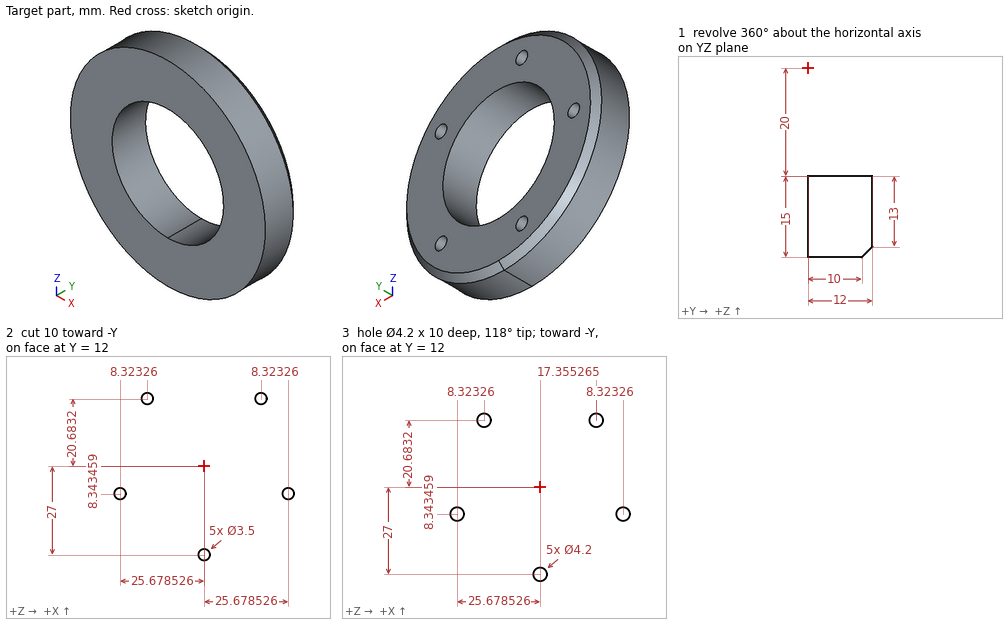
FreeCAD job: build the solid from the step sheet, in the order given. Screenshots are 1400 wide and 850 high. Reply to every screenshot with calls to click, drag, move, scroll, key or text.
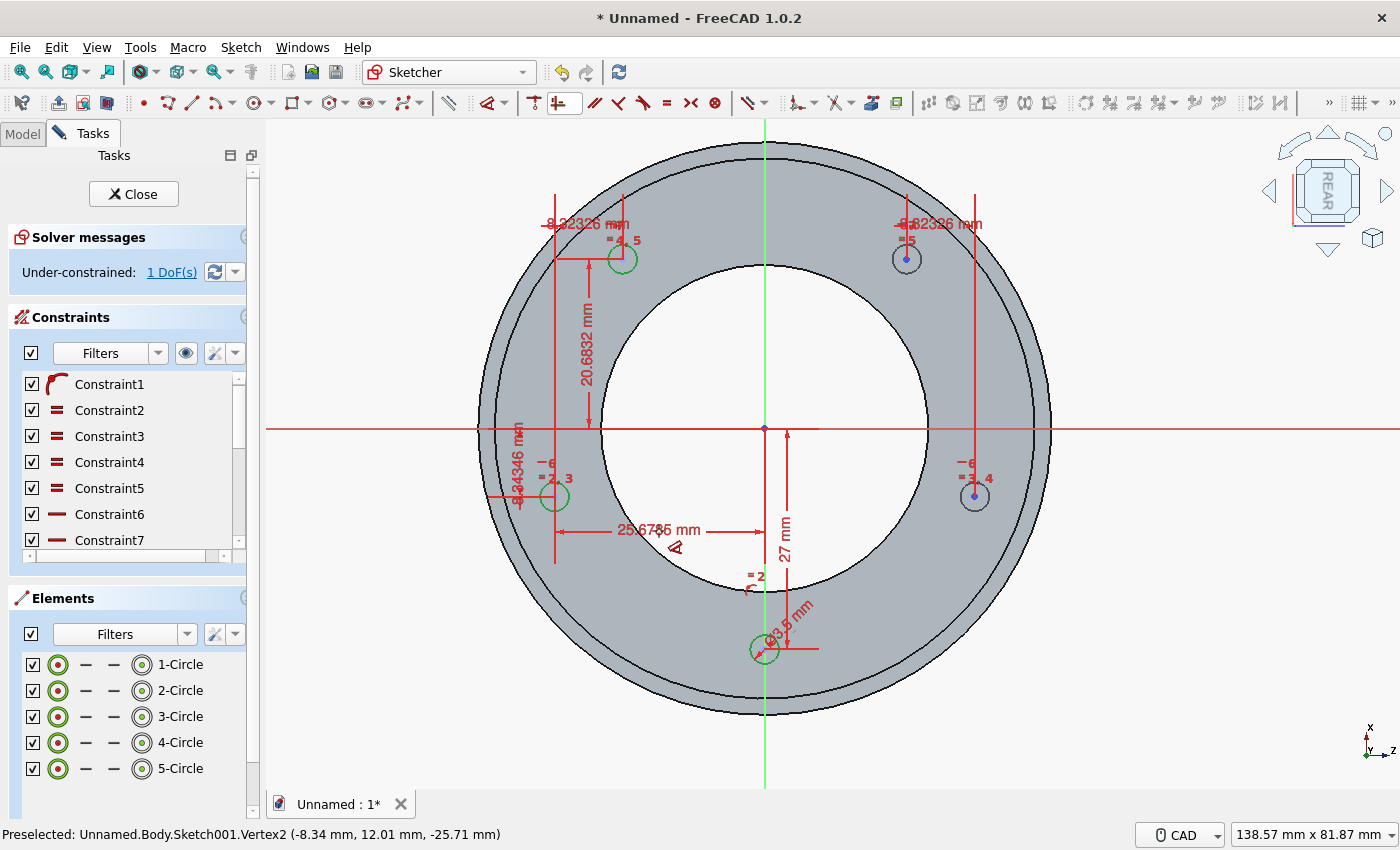
click(975, 497)
click(870, 531)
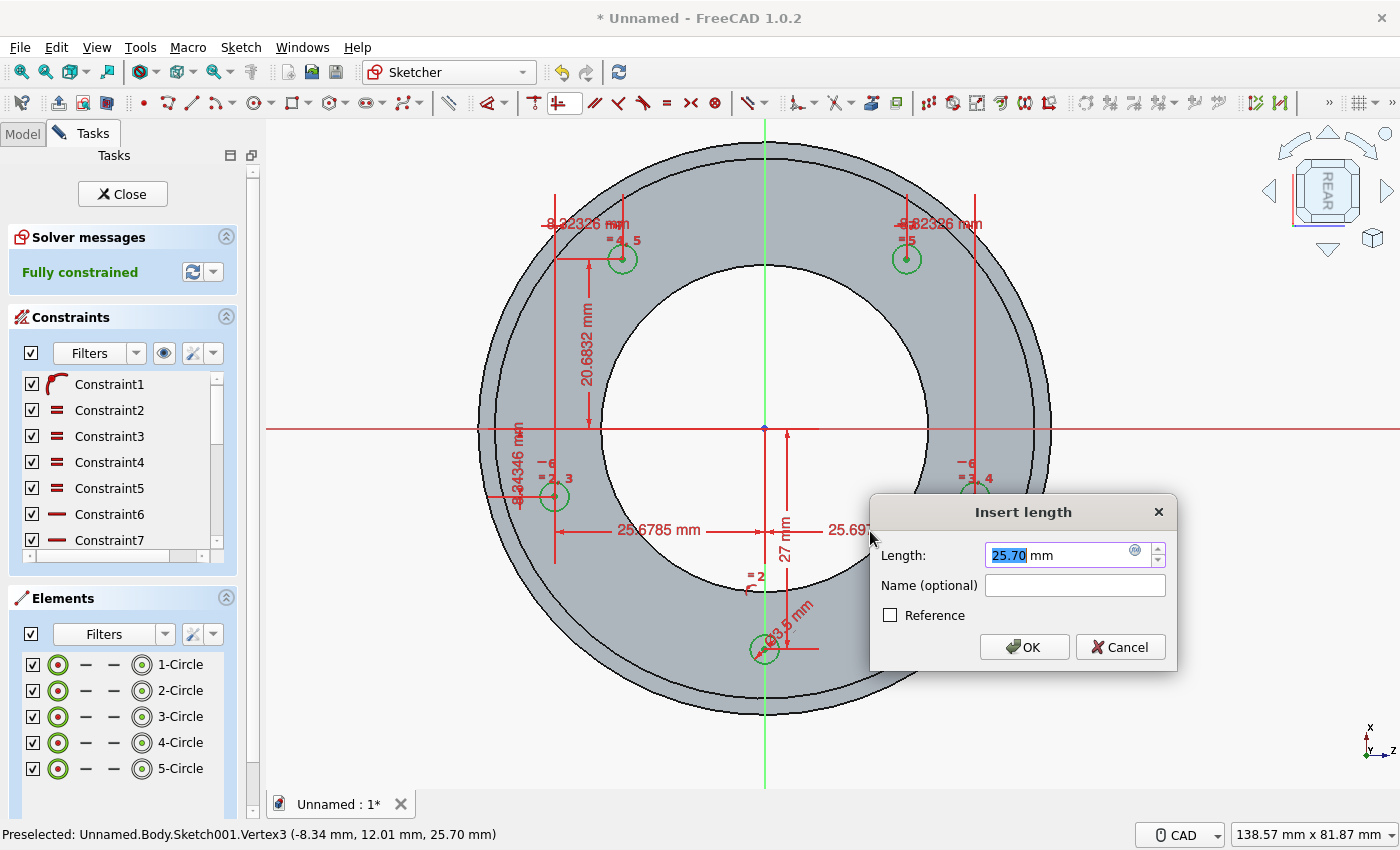
text(25.678526)
key(Return)
key(Escape)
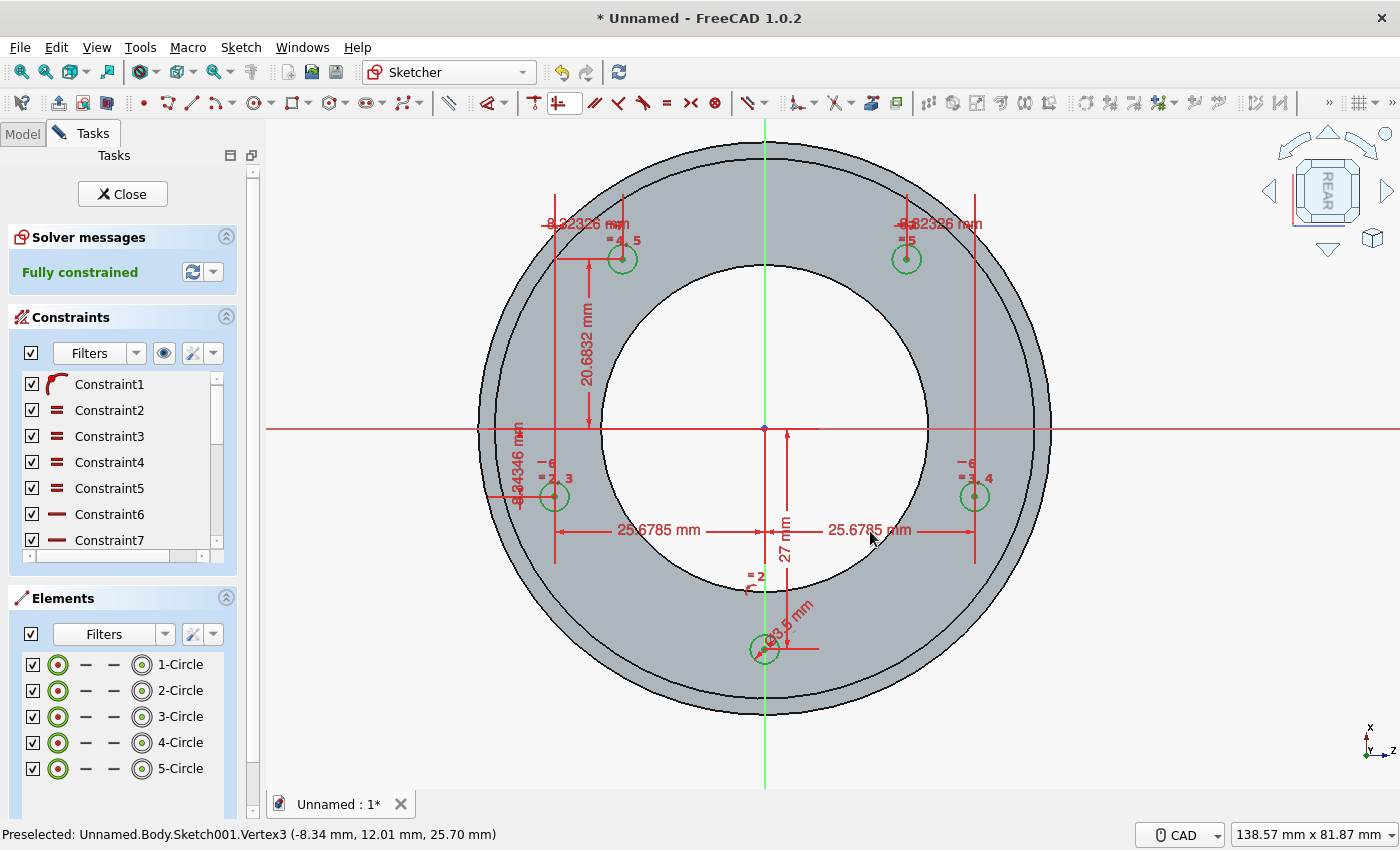
click(123, 194)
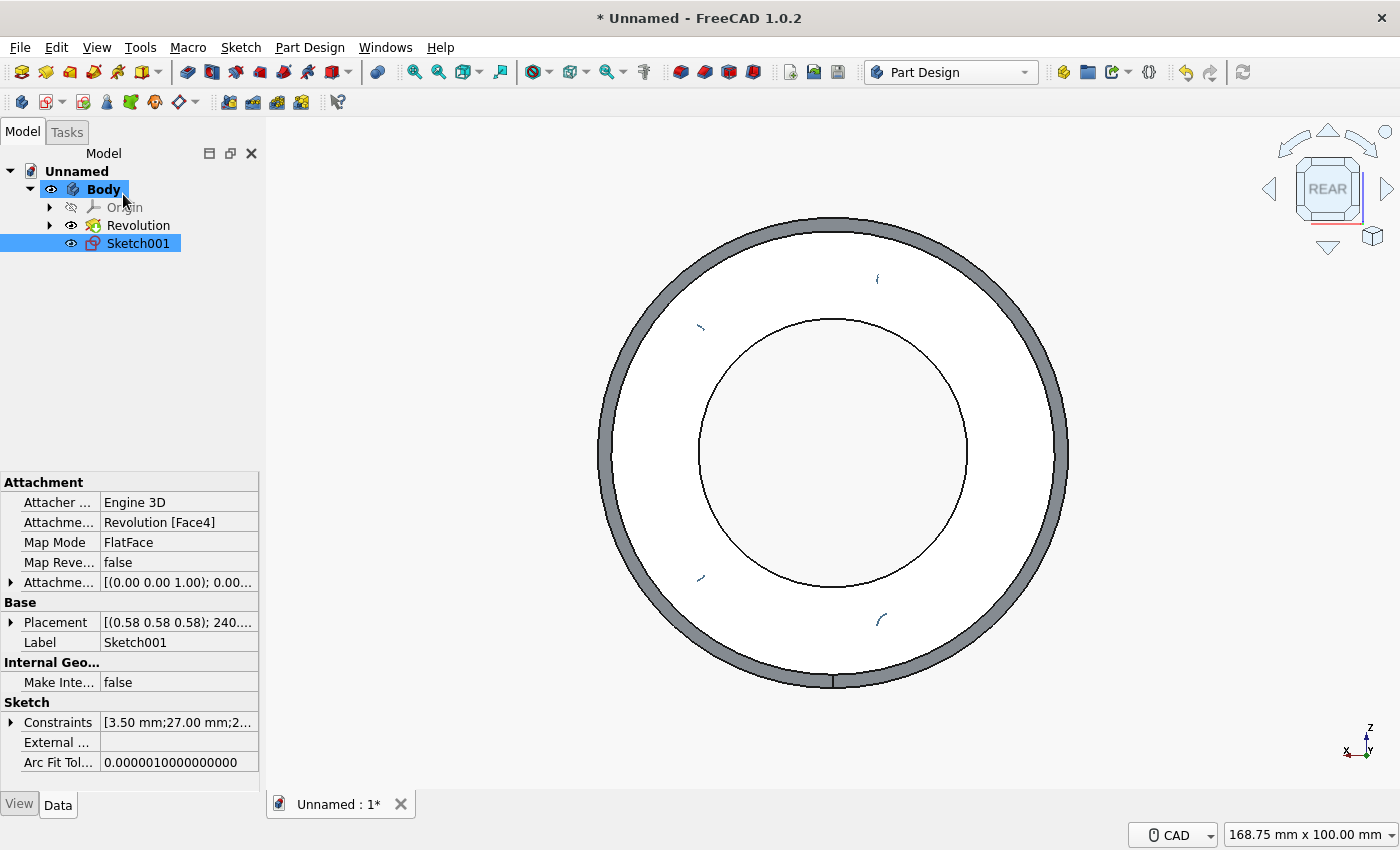
click(188, 72)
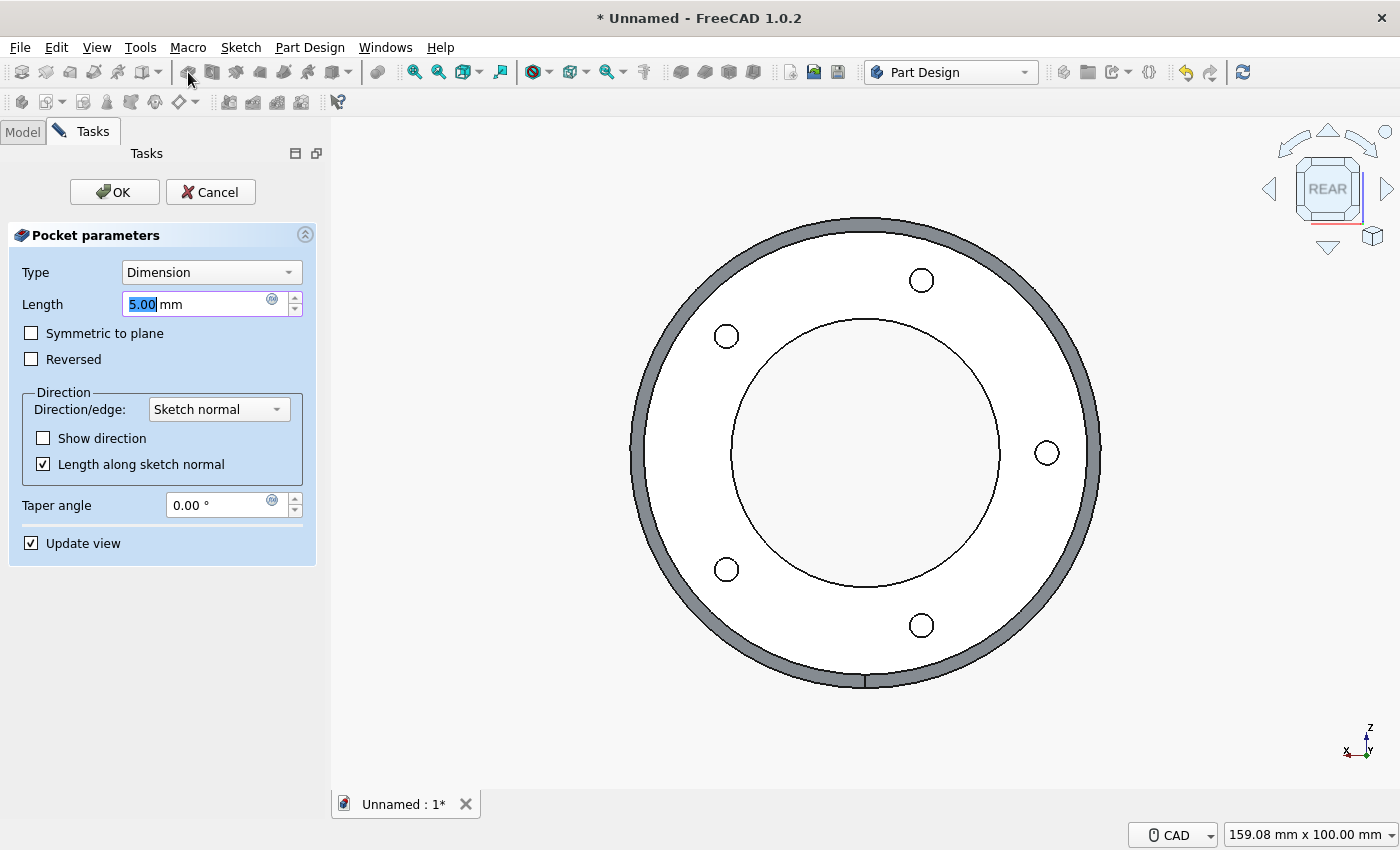
text(10)
key(Tab)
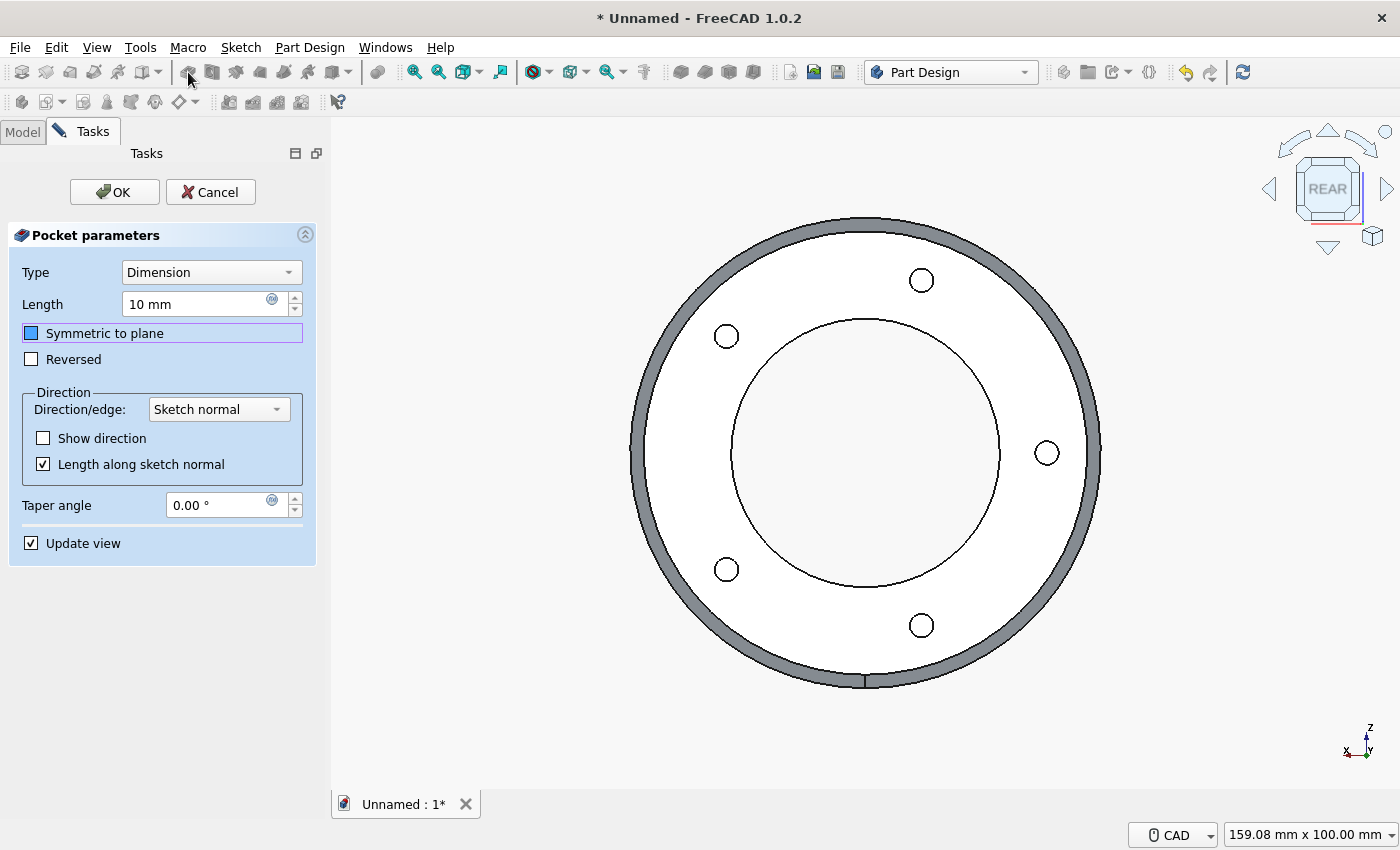
click(115, 192)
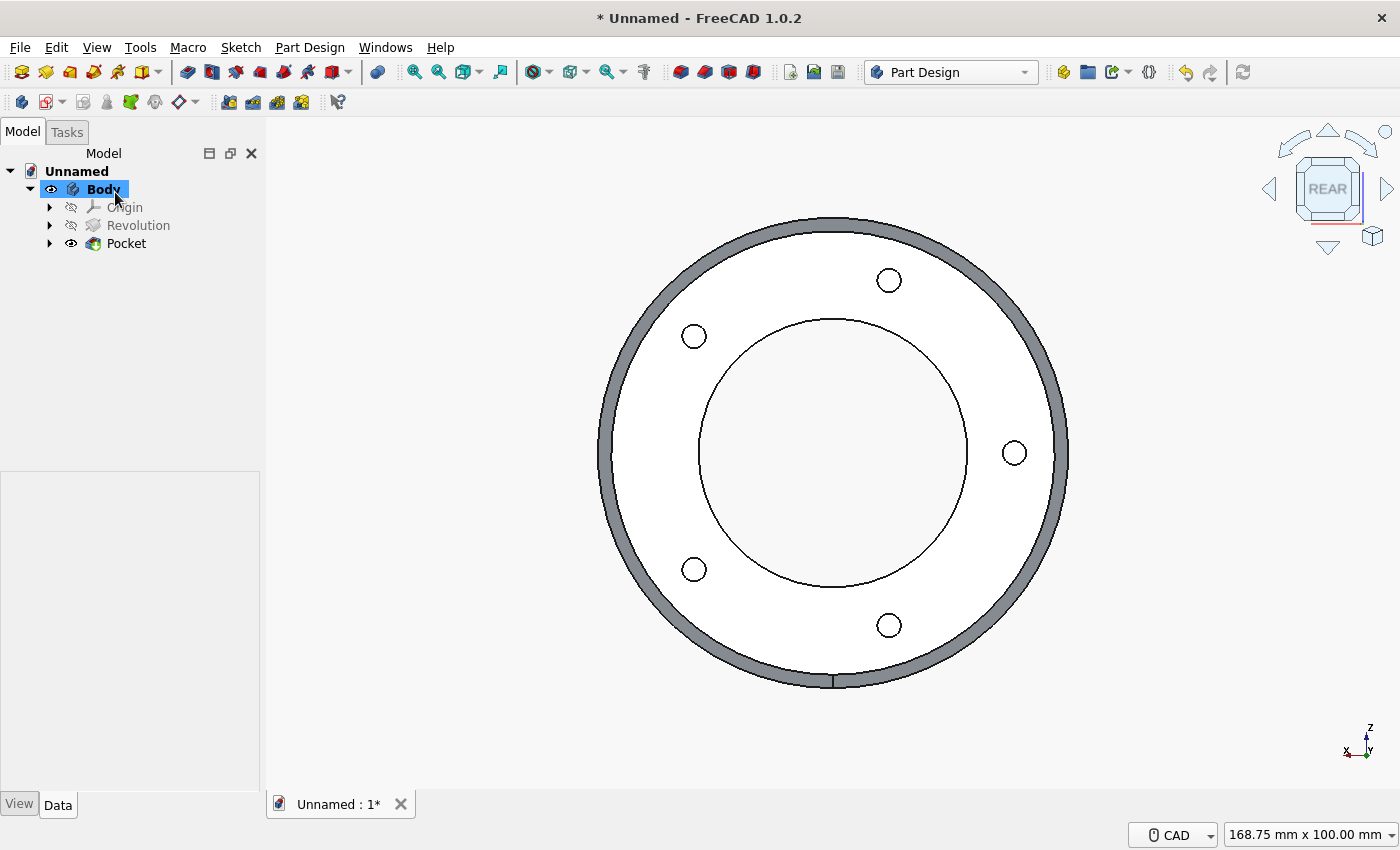
click(960, 325)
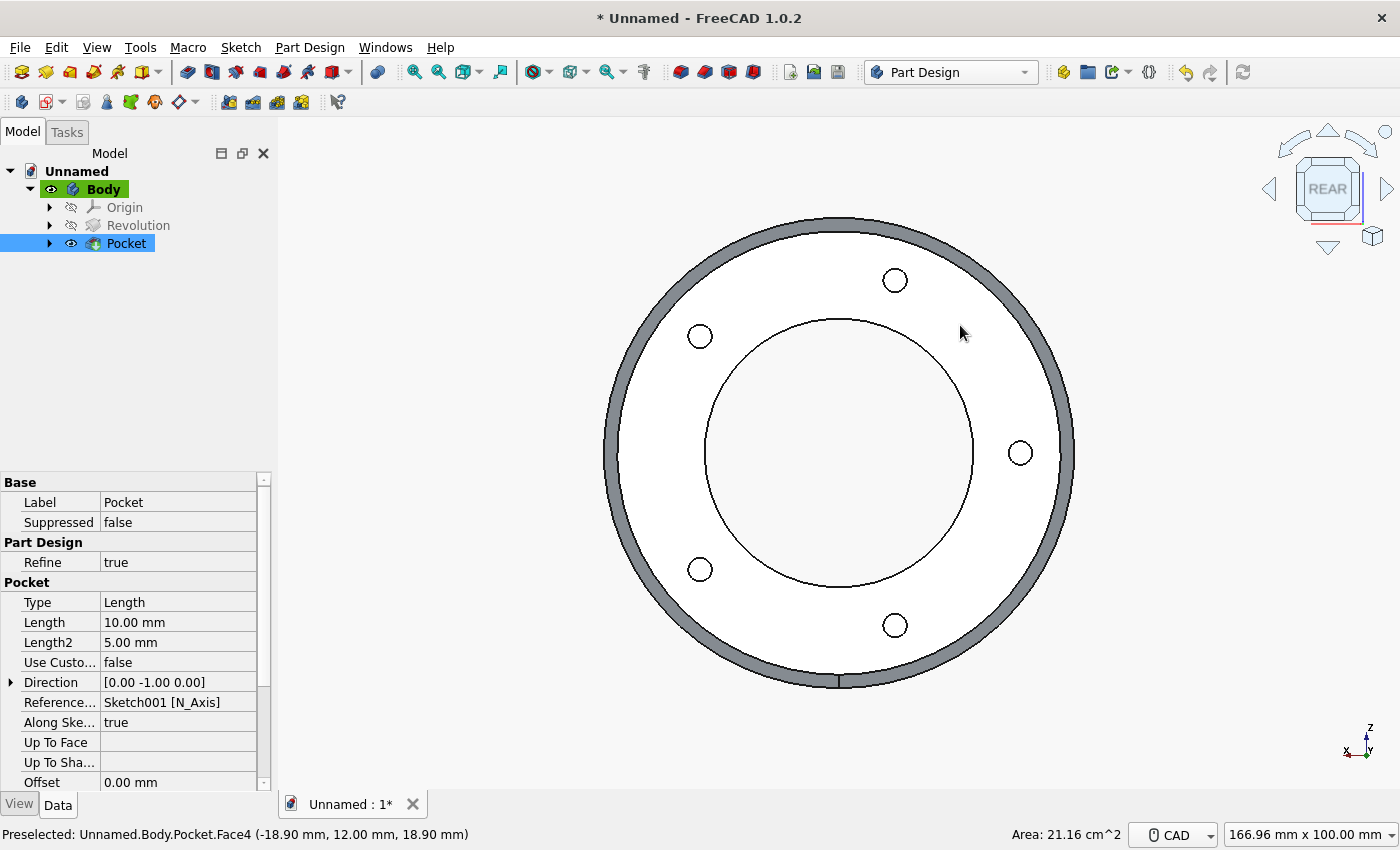
click(46, 102)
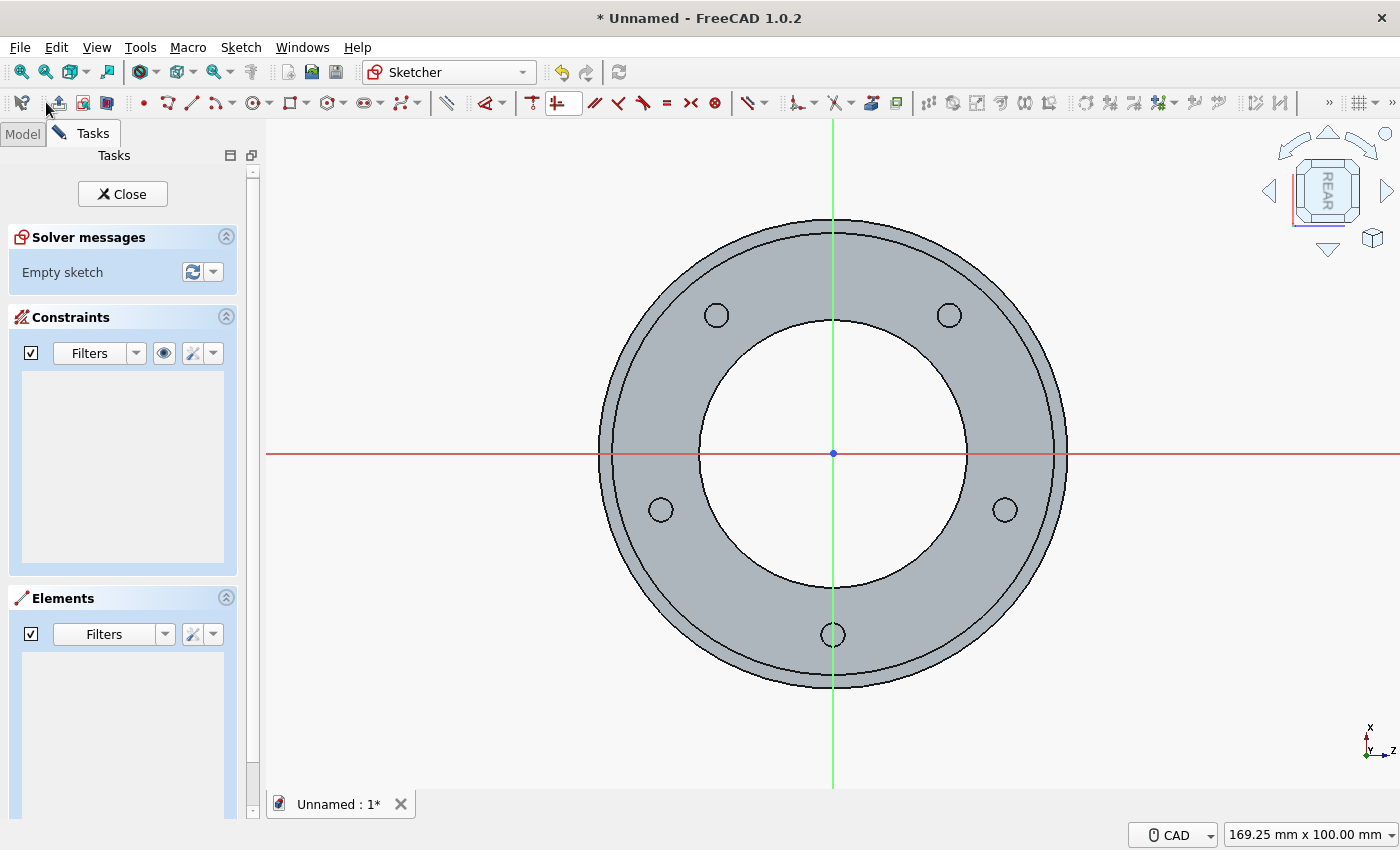
click(254, 104)